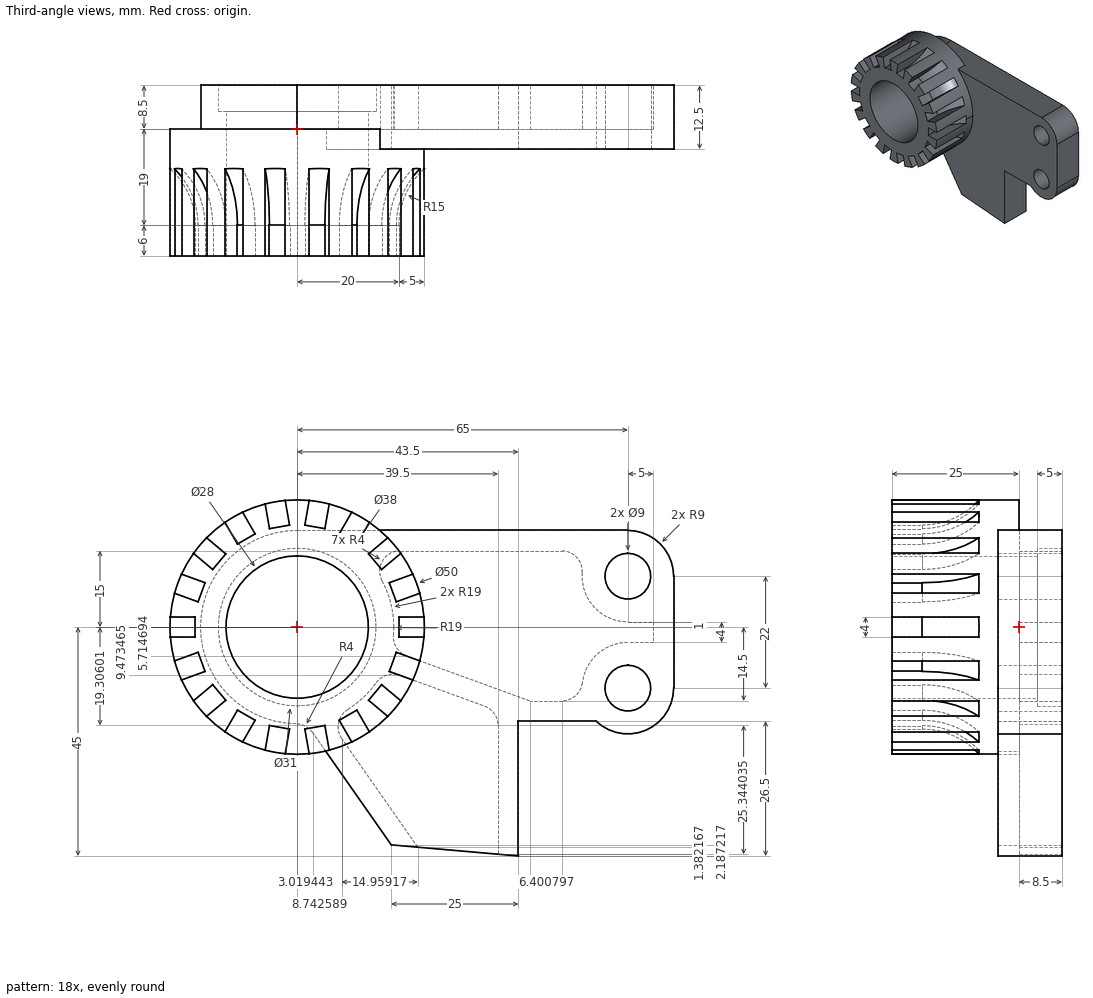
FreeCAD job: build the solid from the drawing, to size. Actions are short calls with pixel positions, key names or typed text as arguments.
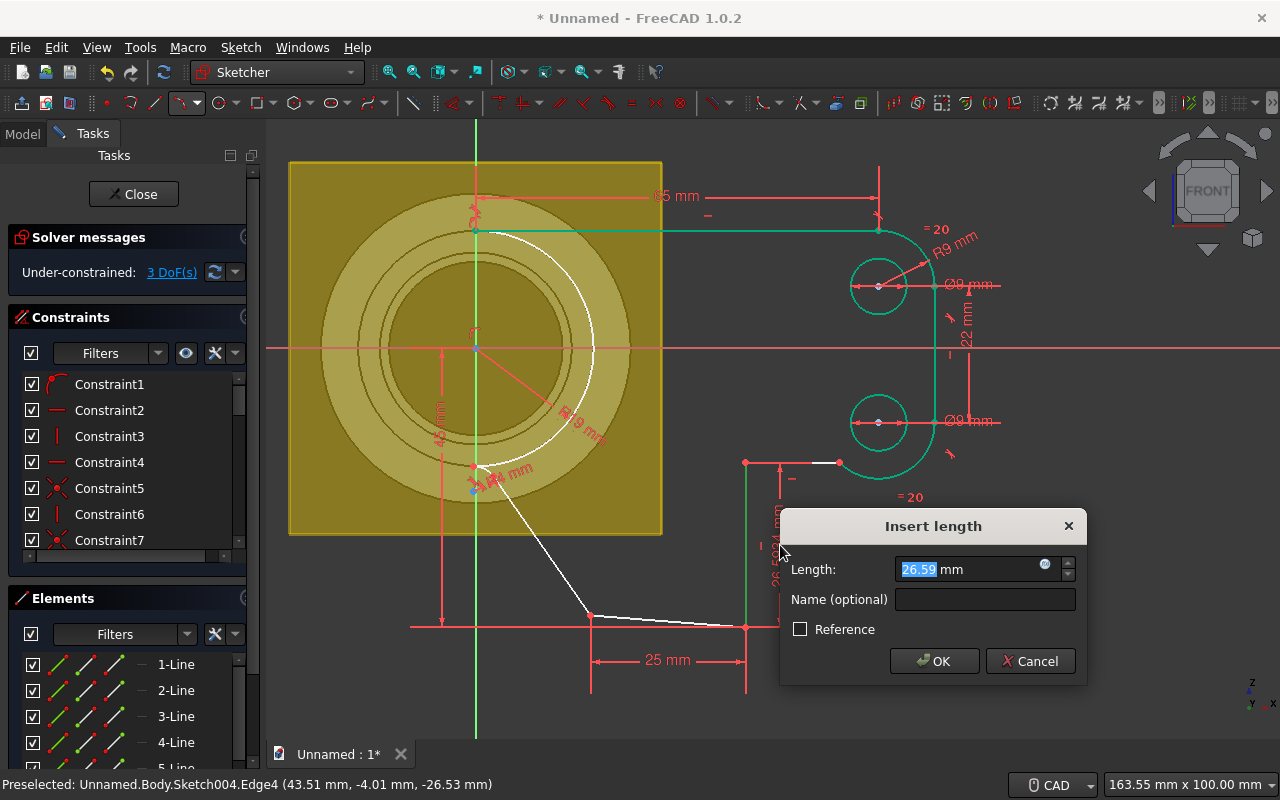
text(26.5)
key(Return)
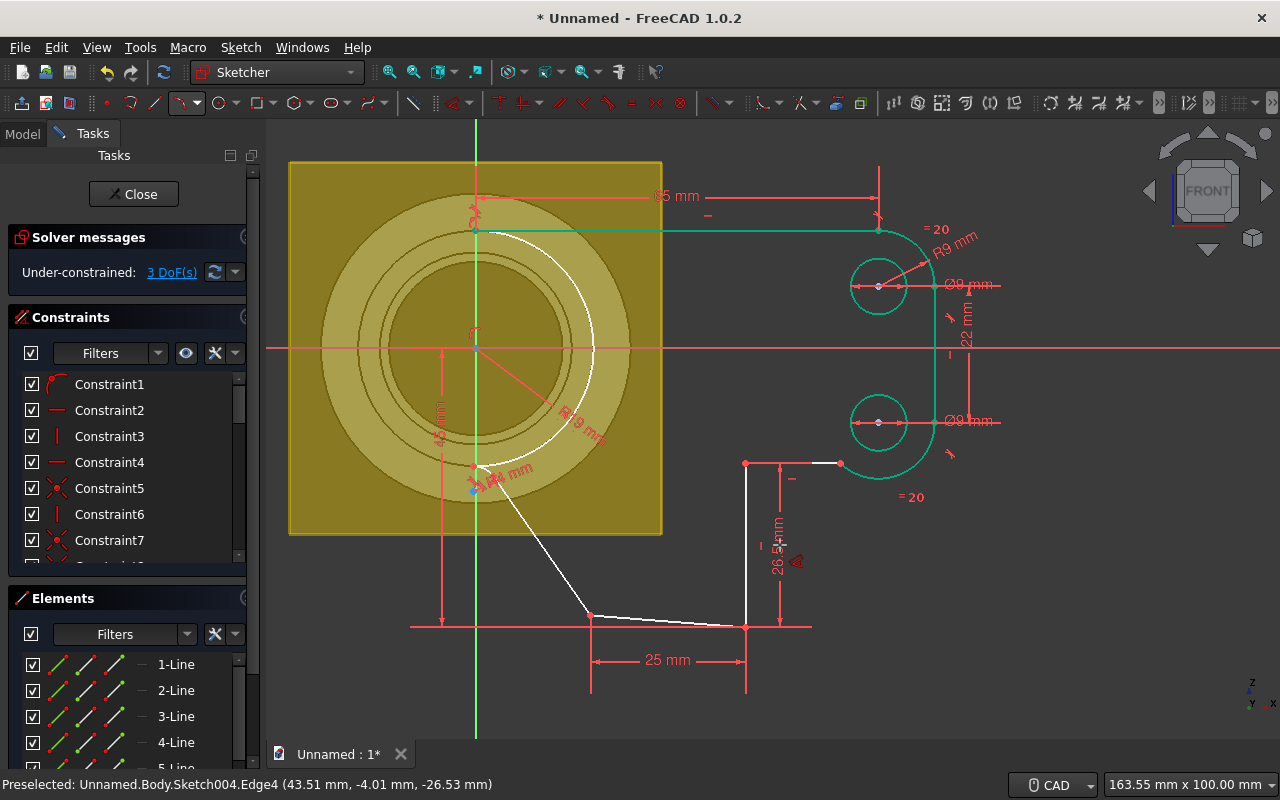
click(746, 463)
click(611, 314)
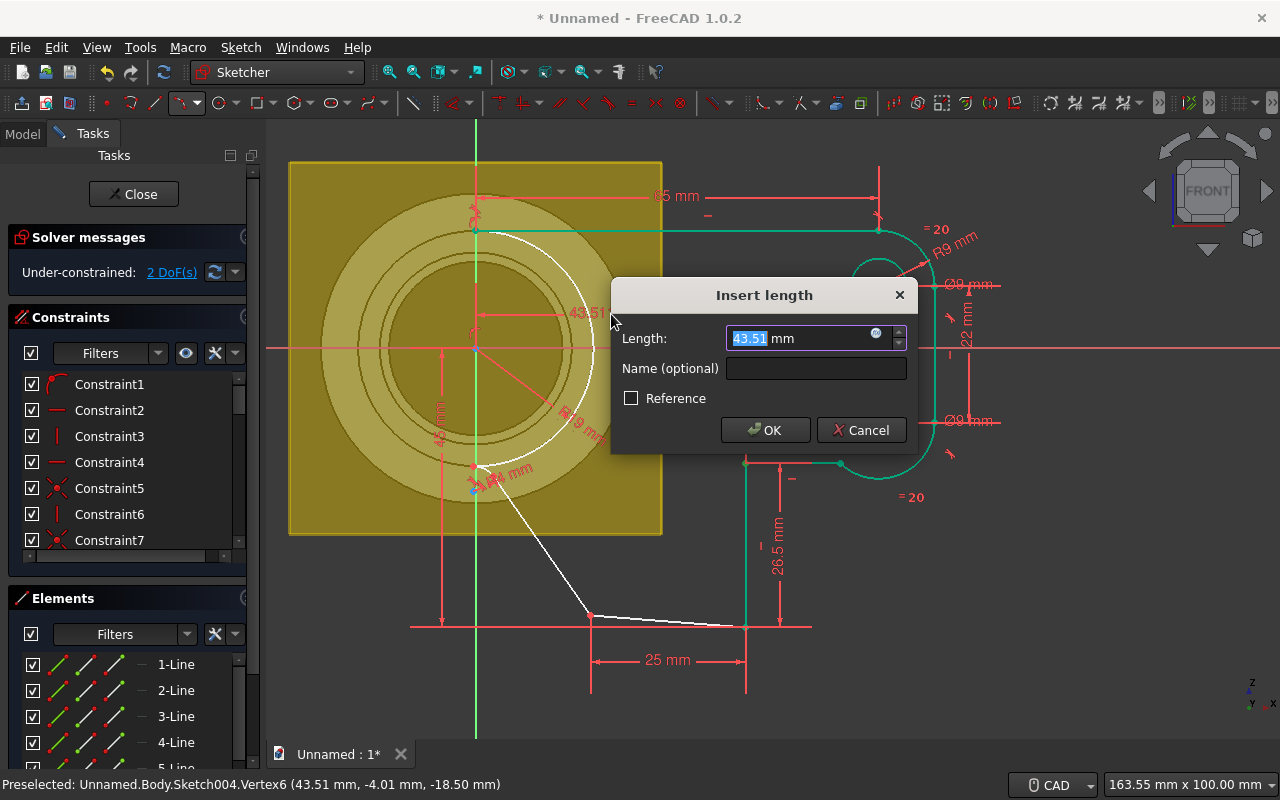
text(43.5)
key(Return)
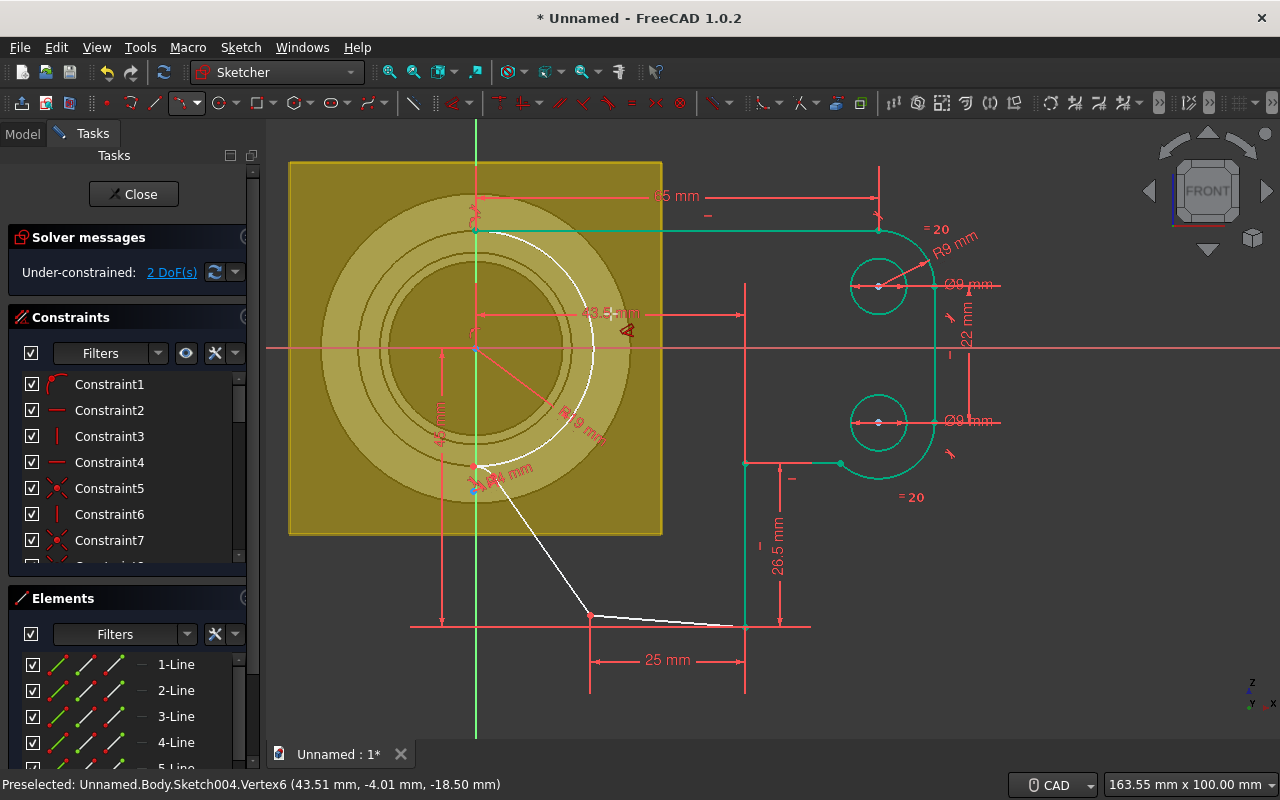
scroll(494, 477, up, 4)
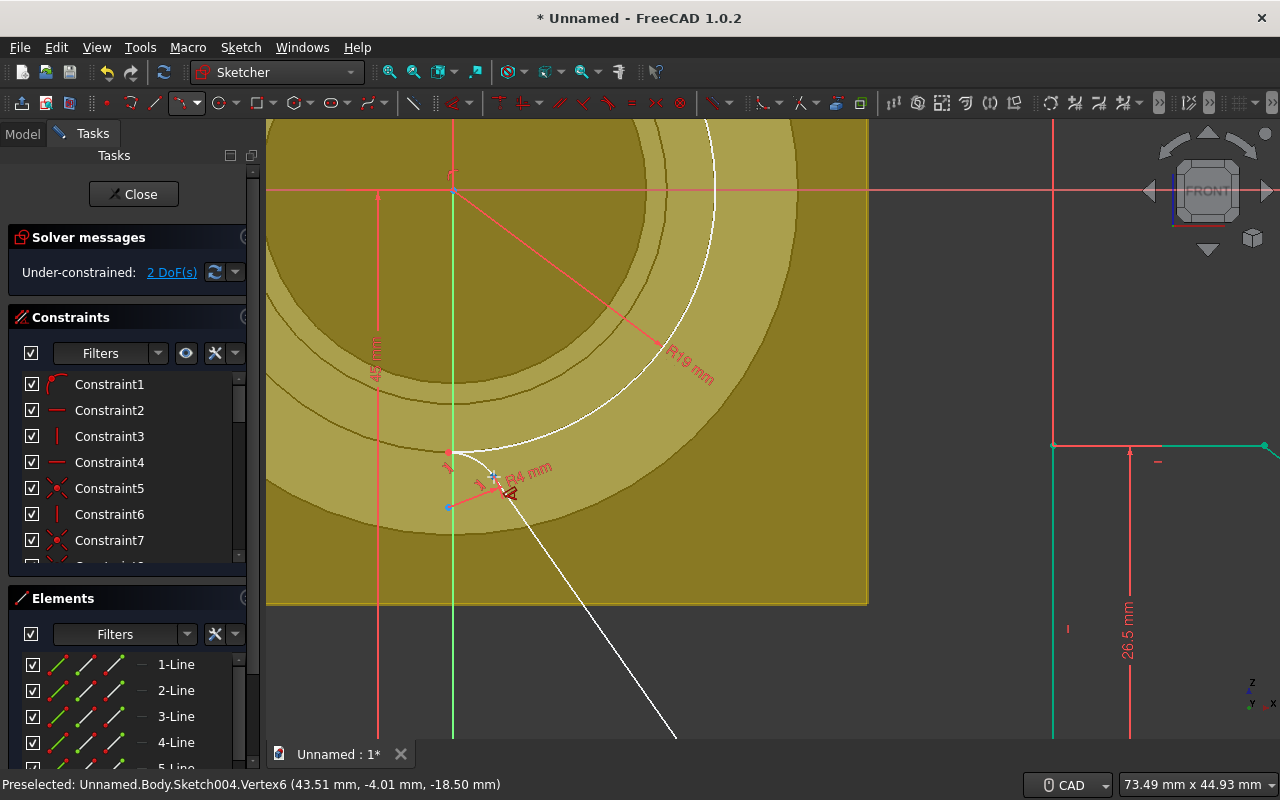
click(493, 476)
click(473, 156)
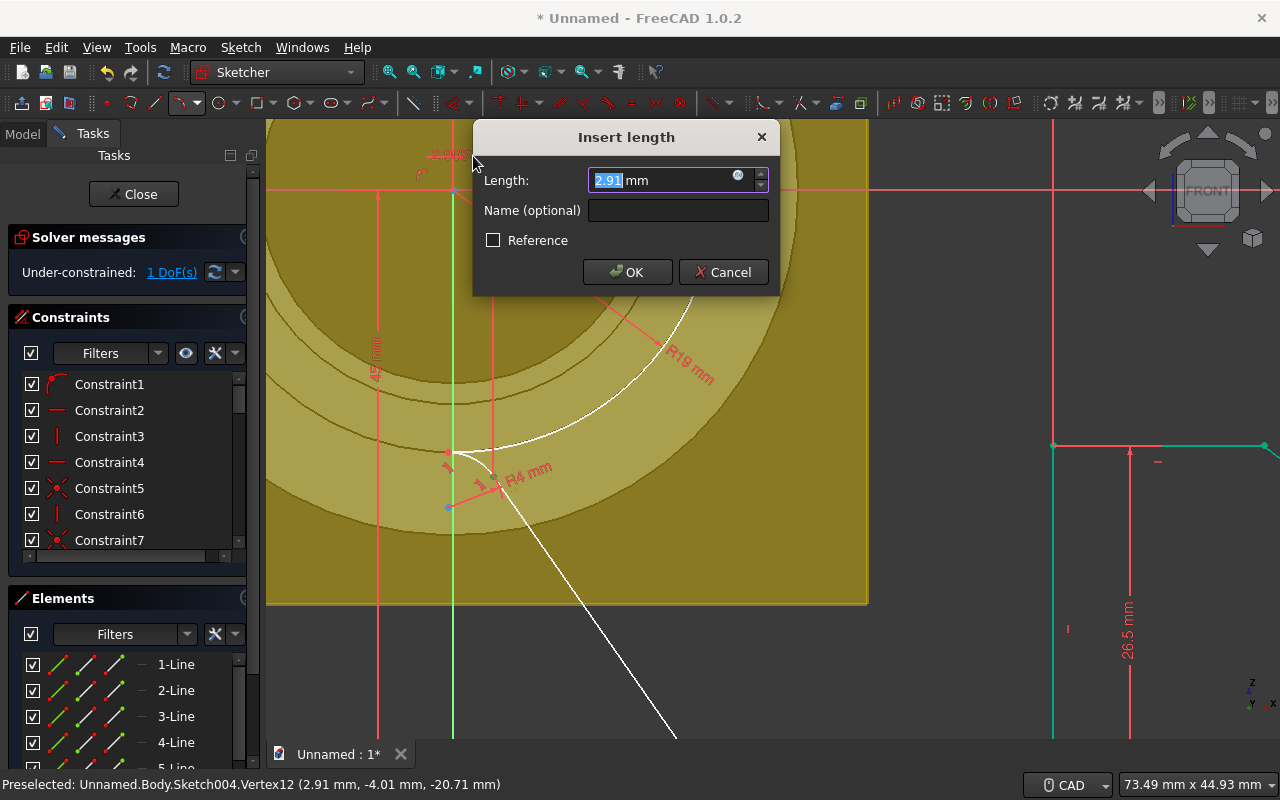
text(3.019443)
key(Return)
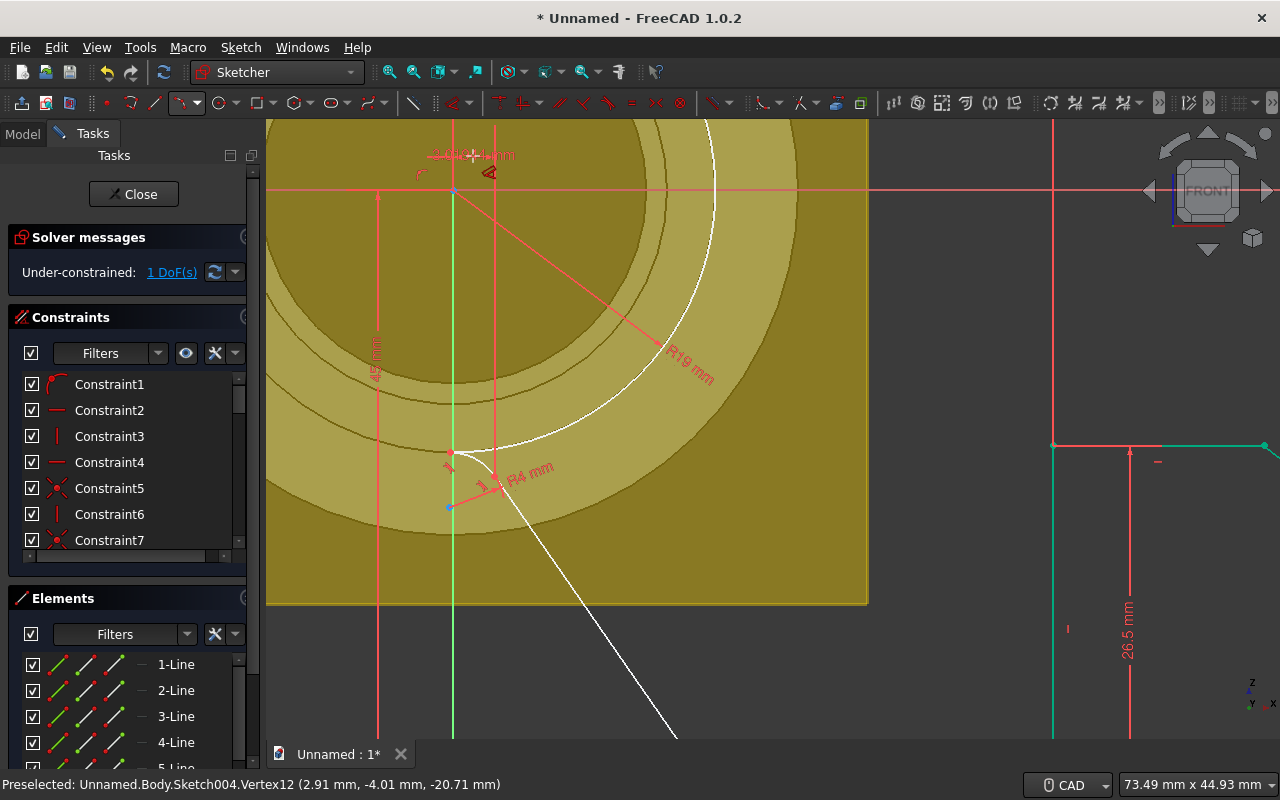
scroll(494, 477, down, 4)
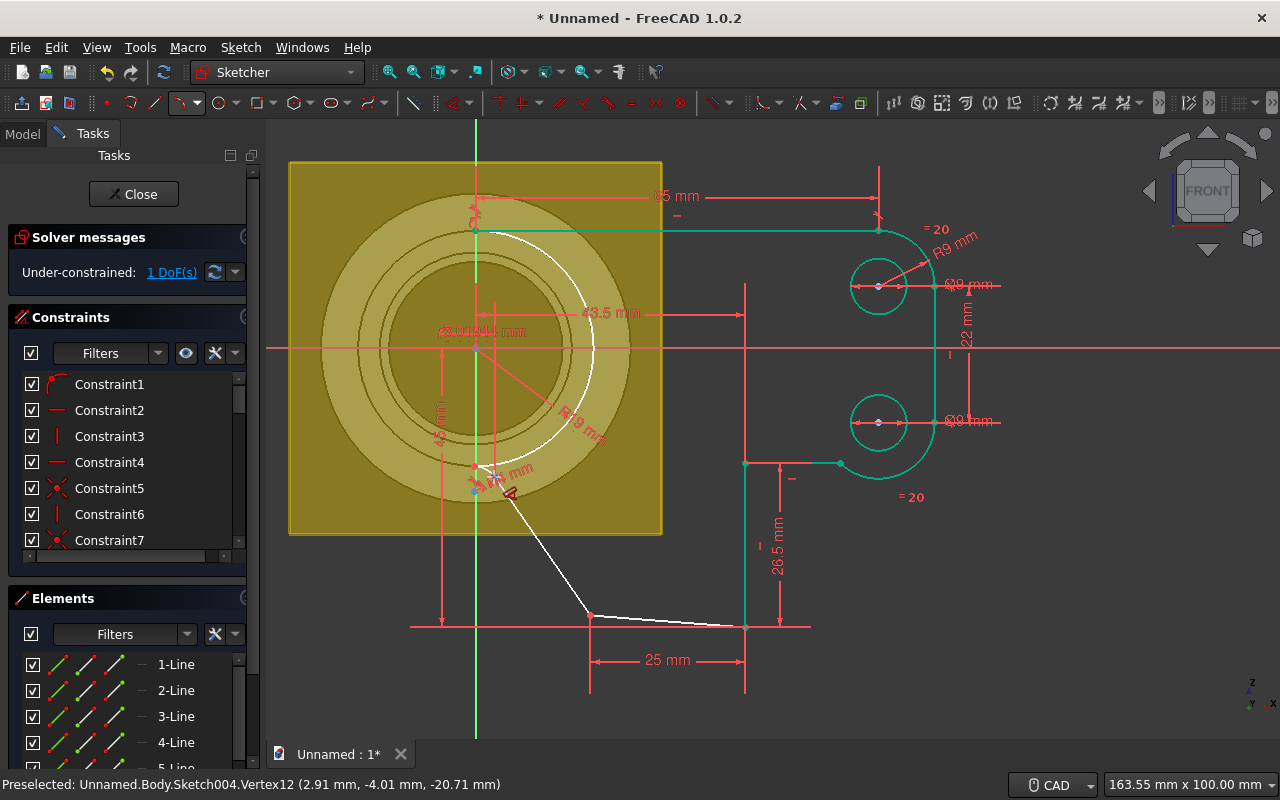
scroll(699, 624, up, 6)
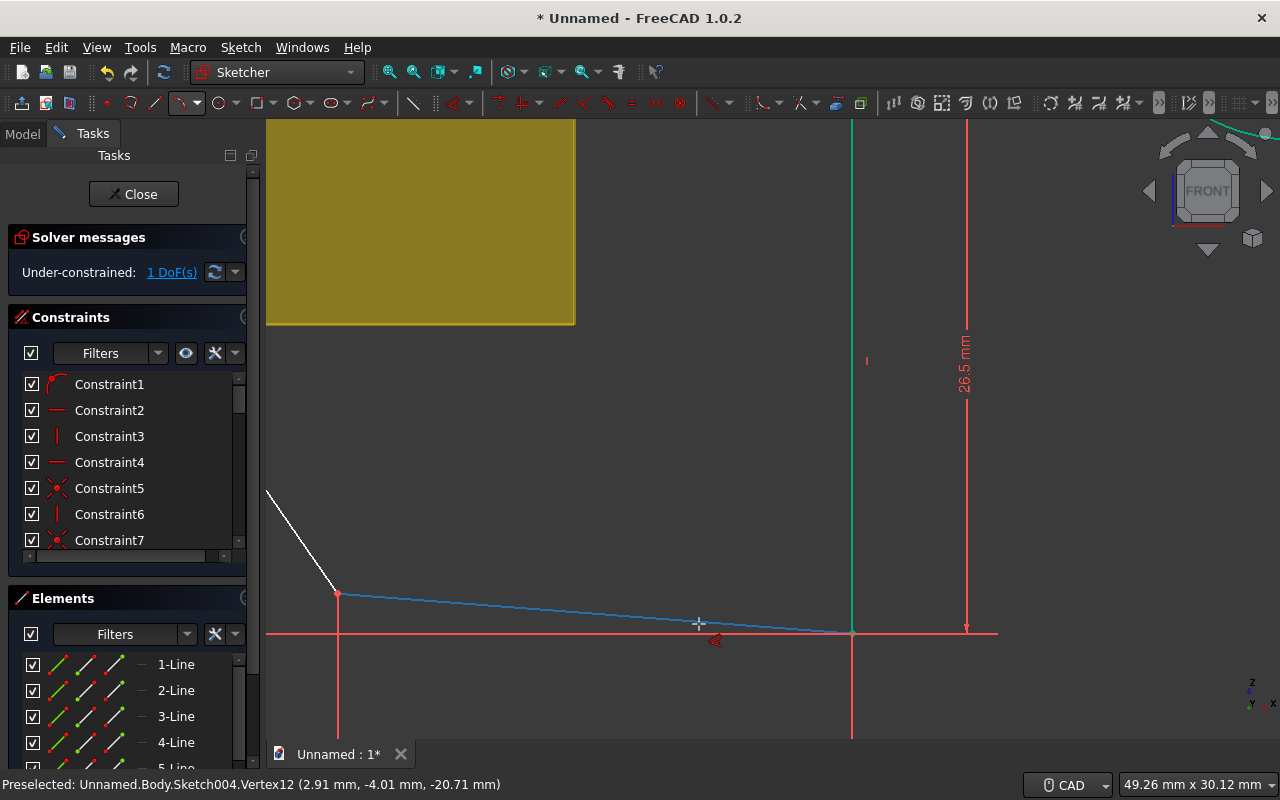
click(698, 622)
click(304, 614)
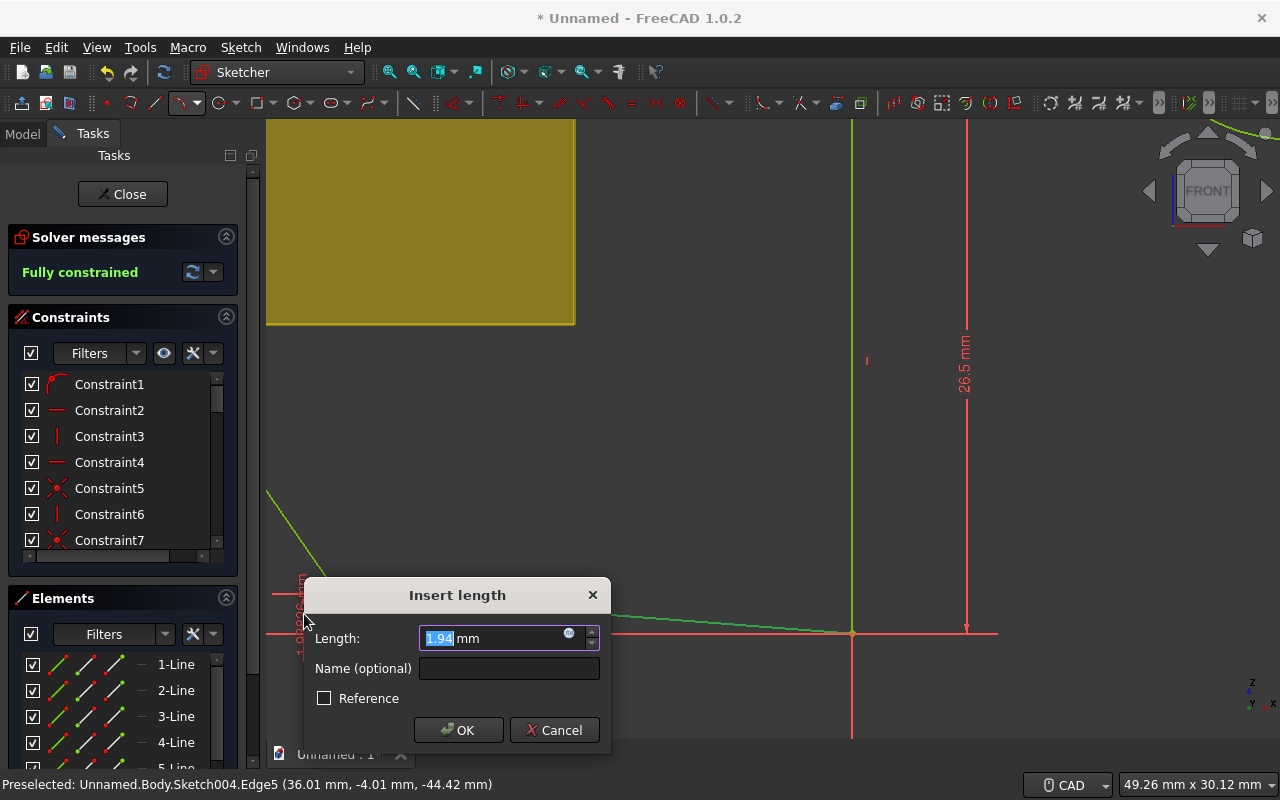
text(2.187217)
key(Return)
key(Escape)